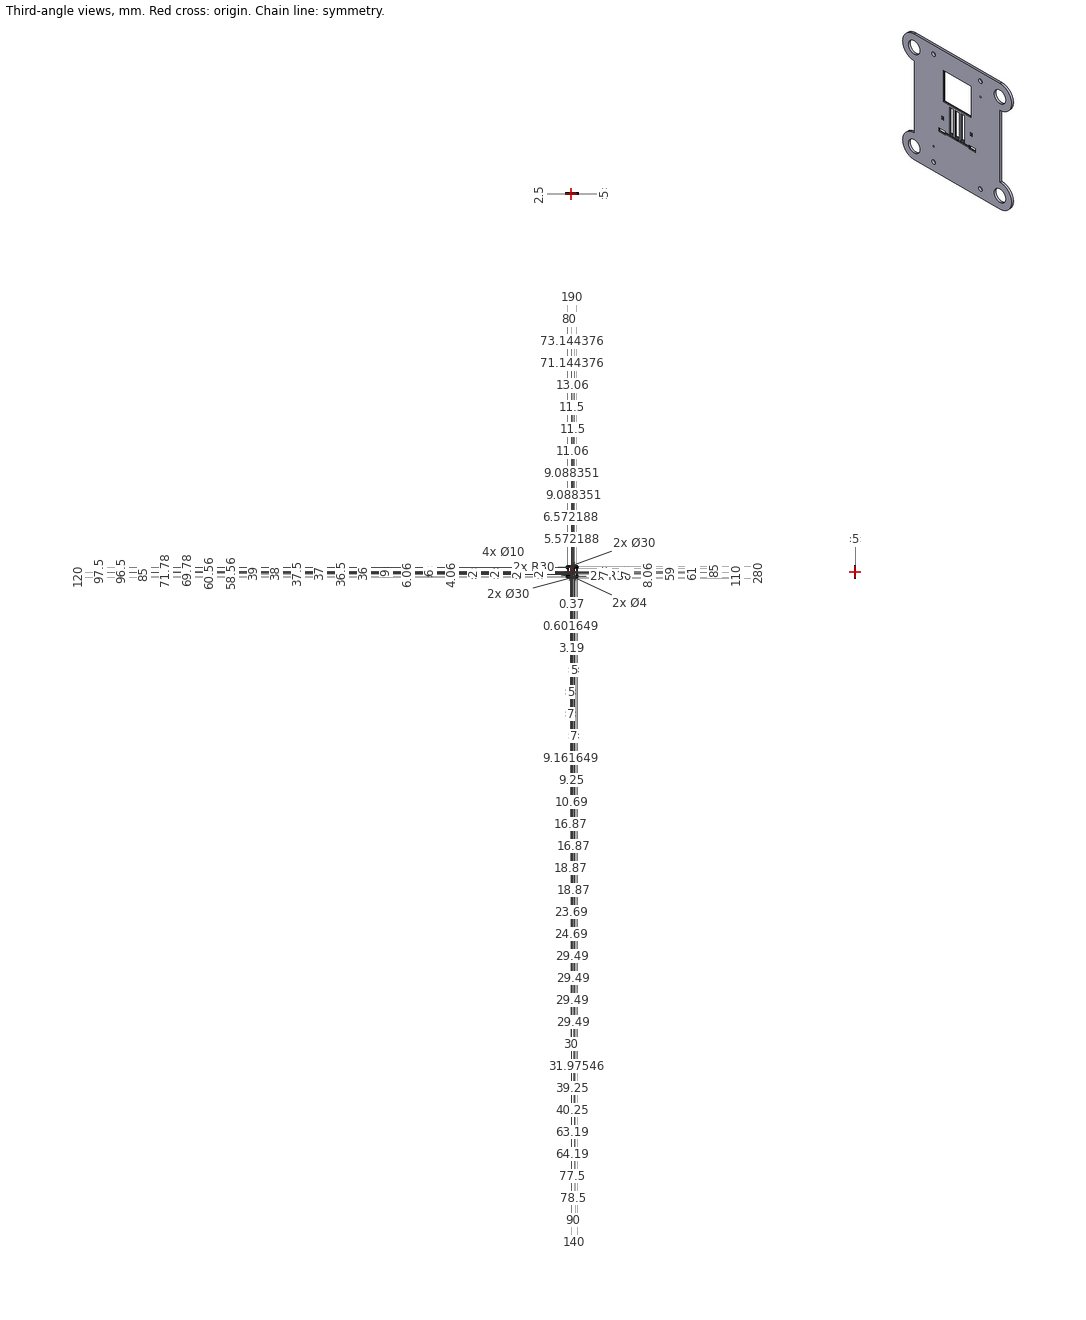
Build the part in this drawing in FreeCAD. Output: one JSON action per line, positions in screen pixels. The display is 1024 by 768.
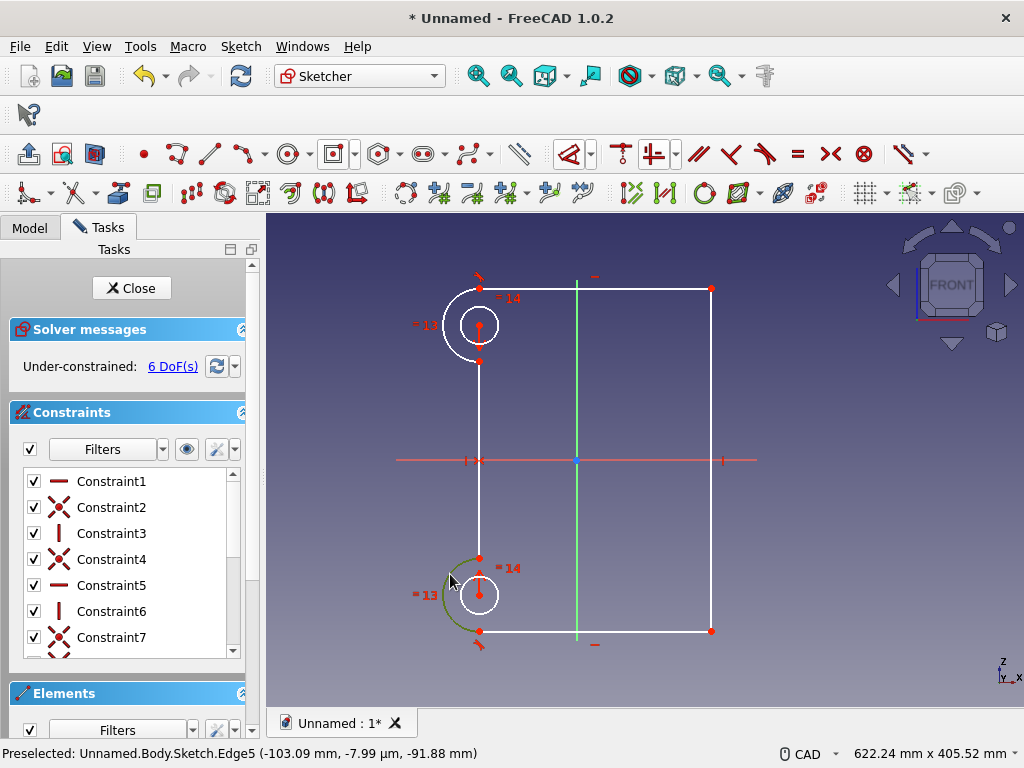
{"action": "key", "text": "k r"}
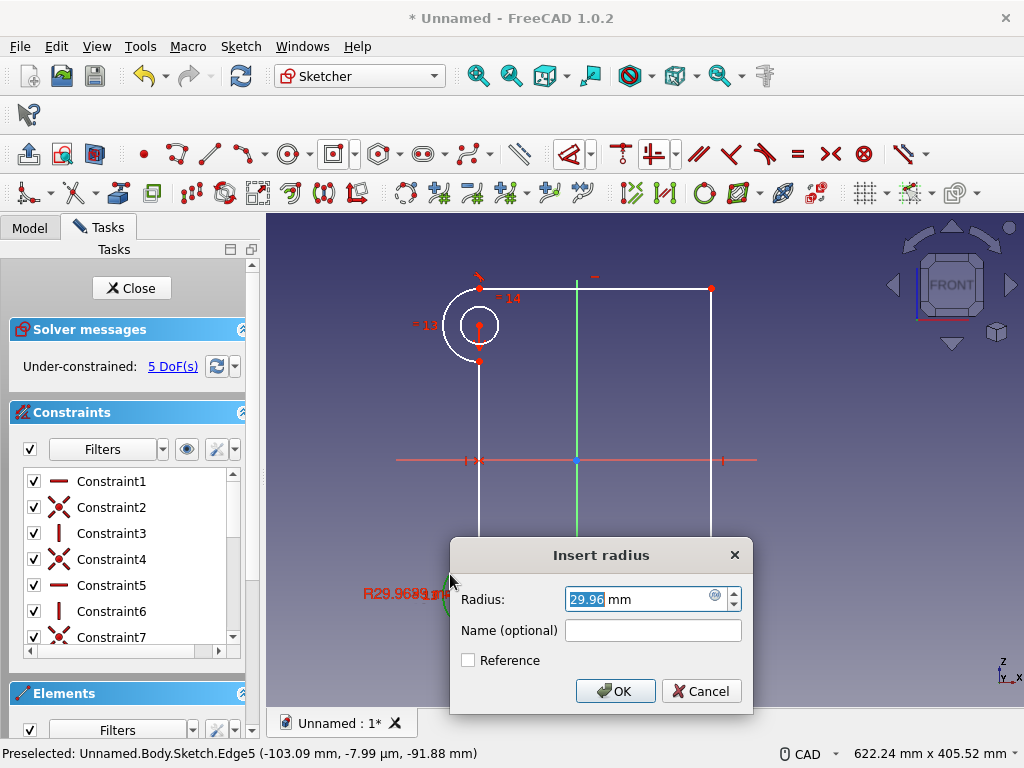
{"action": "type", "text": "30"}
{"action": "key", "text": "Return"}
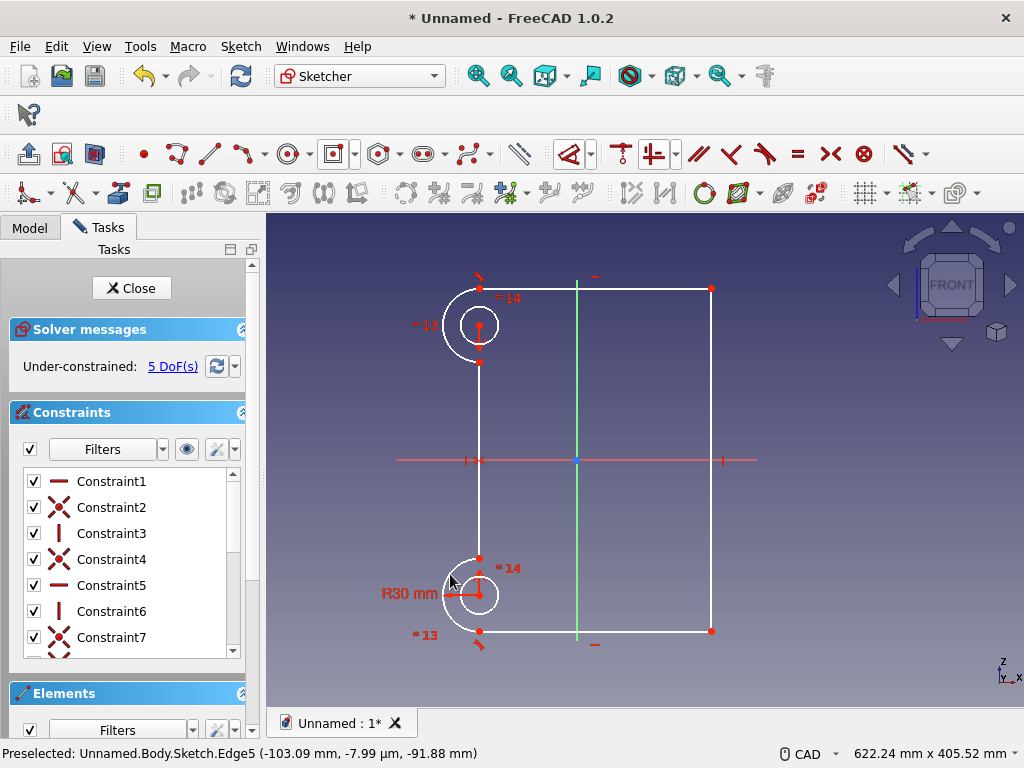
{"action": "left_click", "coordinate": [493, 312]}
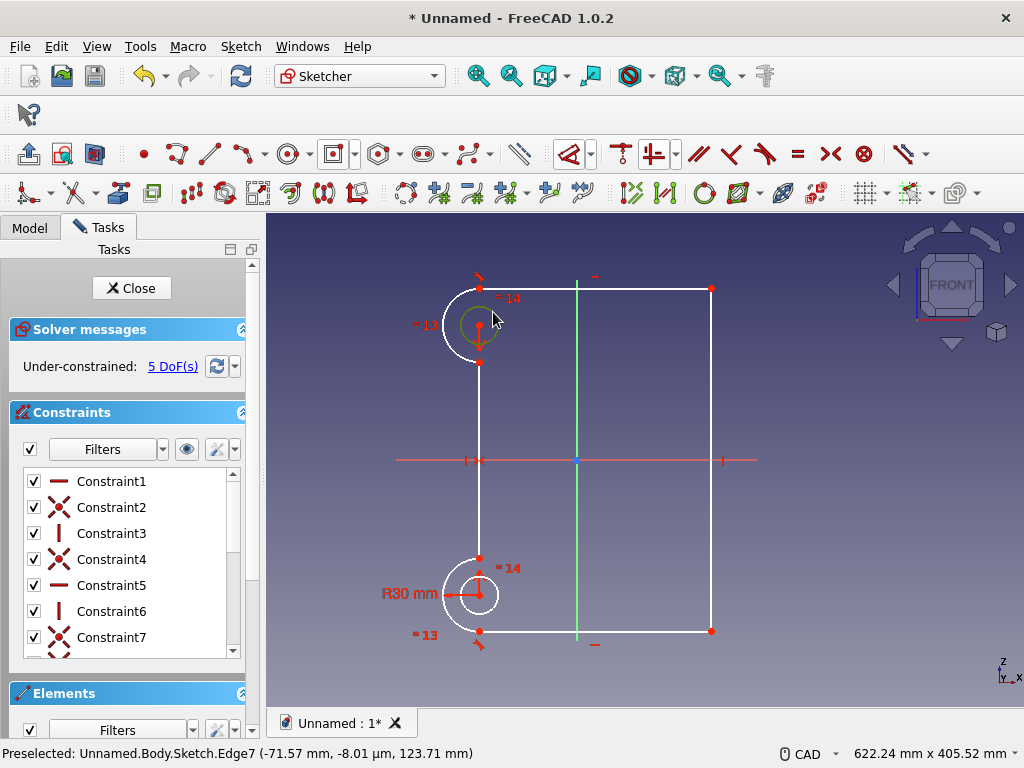
{"action": "key", "text": "k o"}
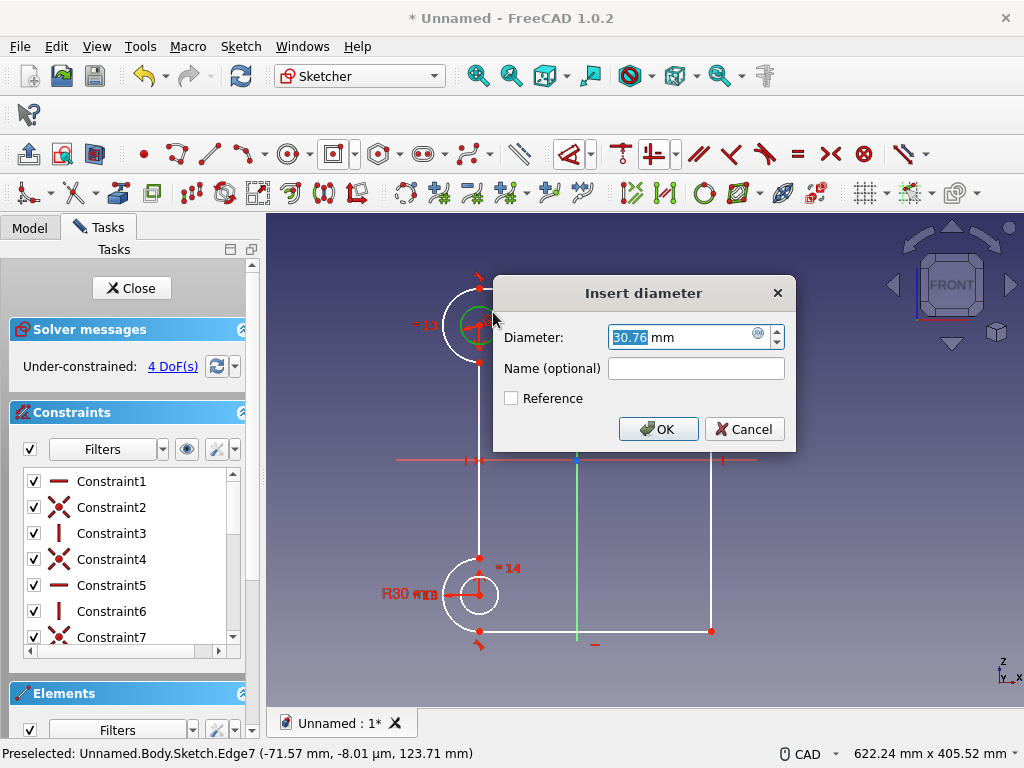
{"action": "type", "text": "30"}
{"action": "key", "text": "Return"}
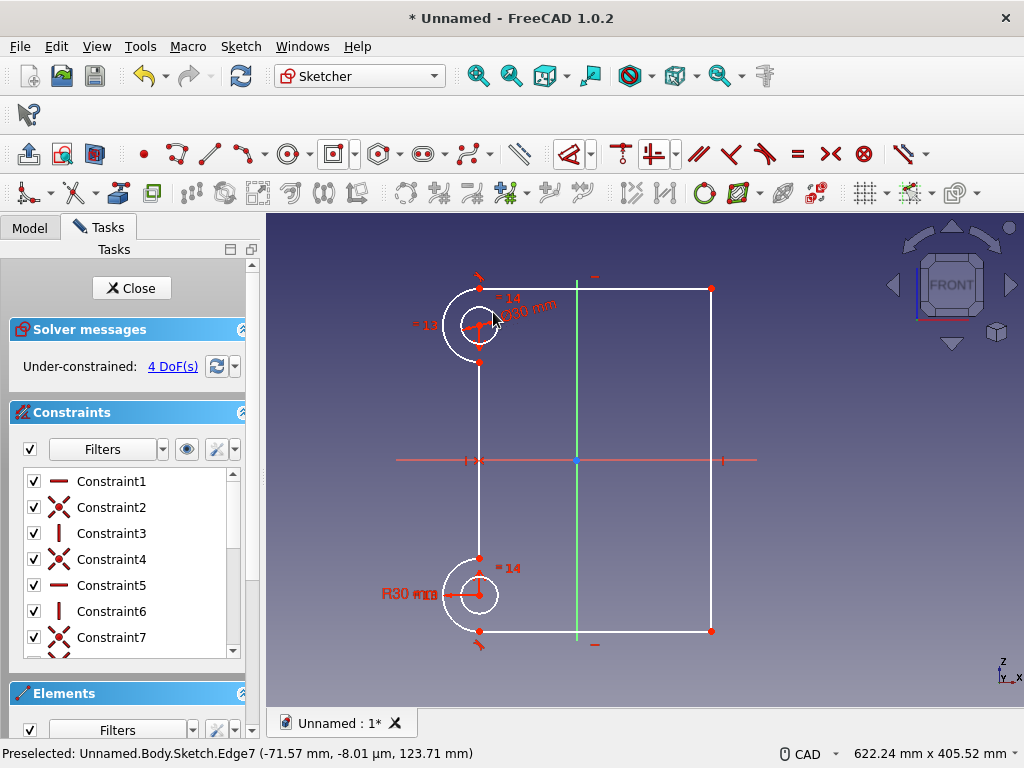
{"action": "left_click", "coordinate": [479, 325]}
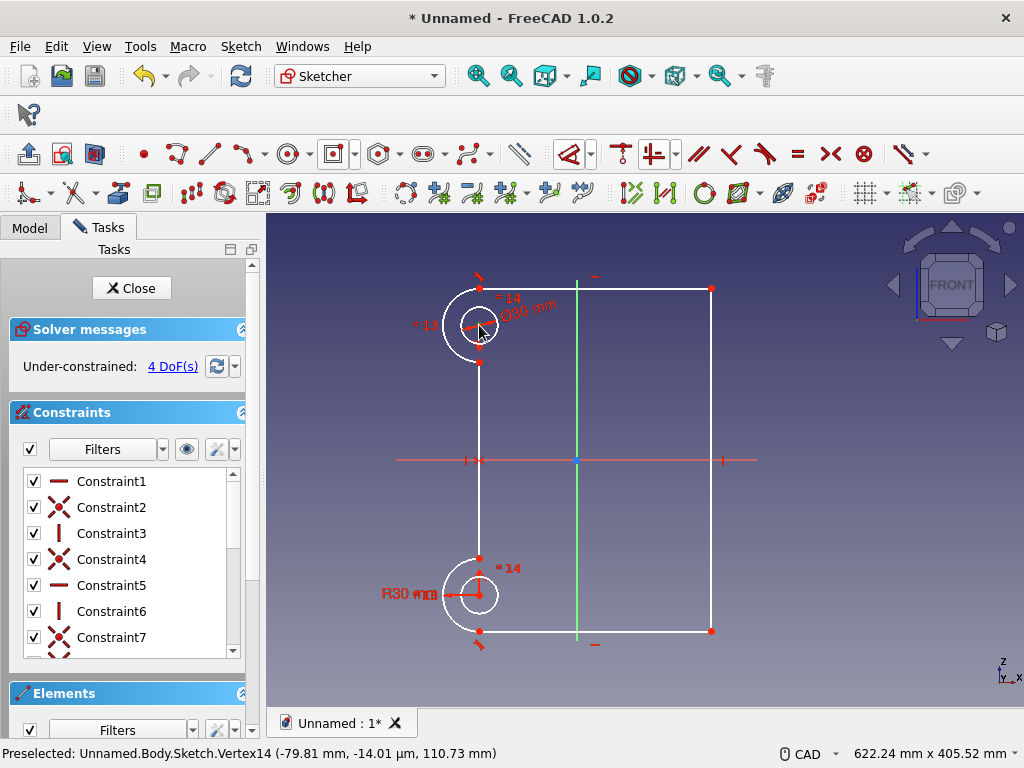
{"action": "key", "text": "l"}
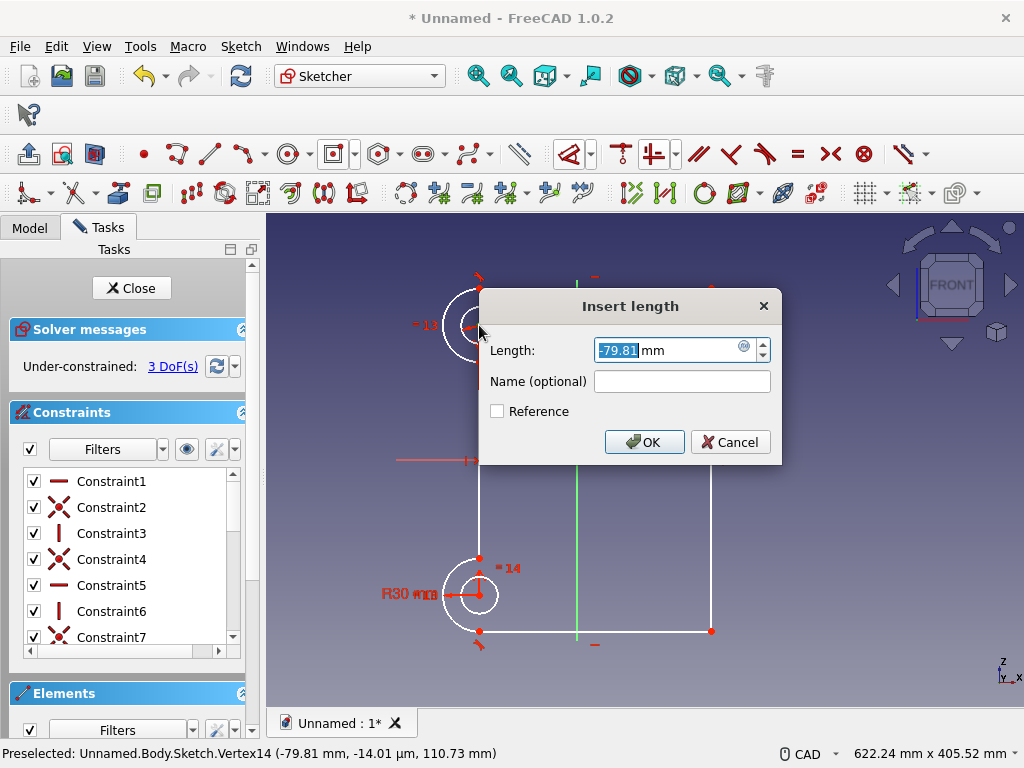
{"action": "type", "text": "-80"}
{"action": "key", "text": "Return"}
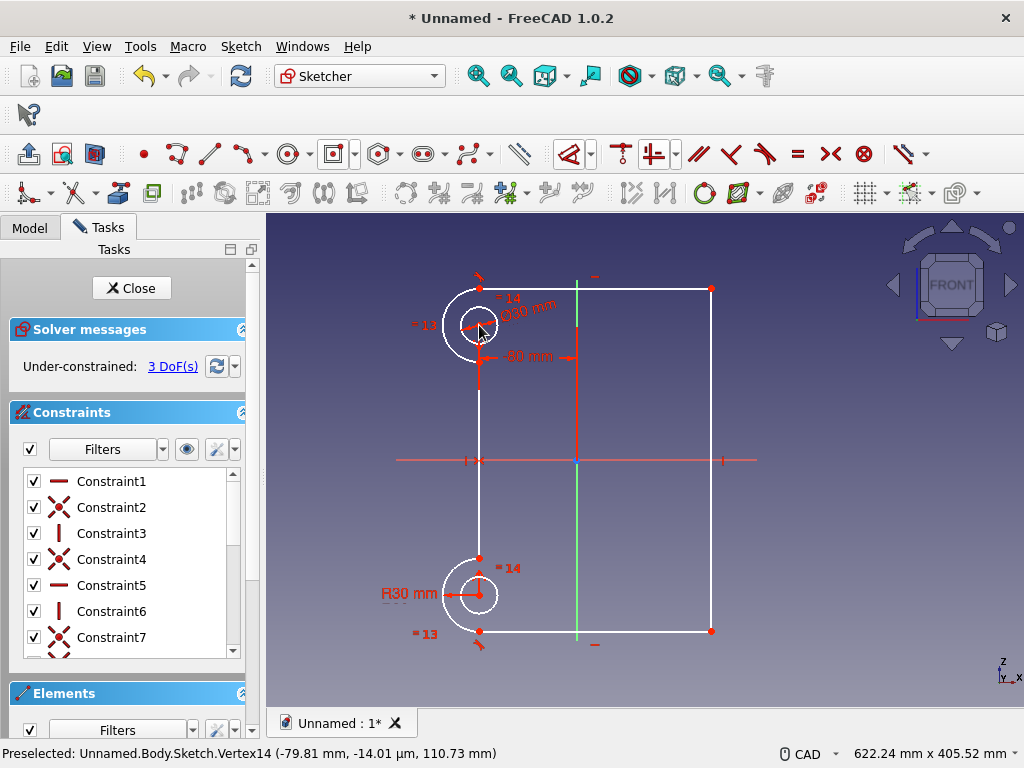
{"action": "left_click", "coordinate": [549, 289]}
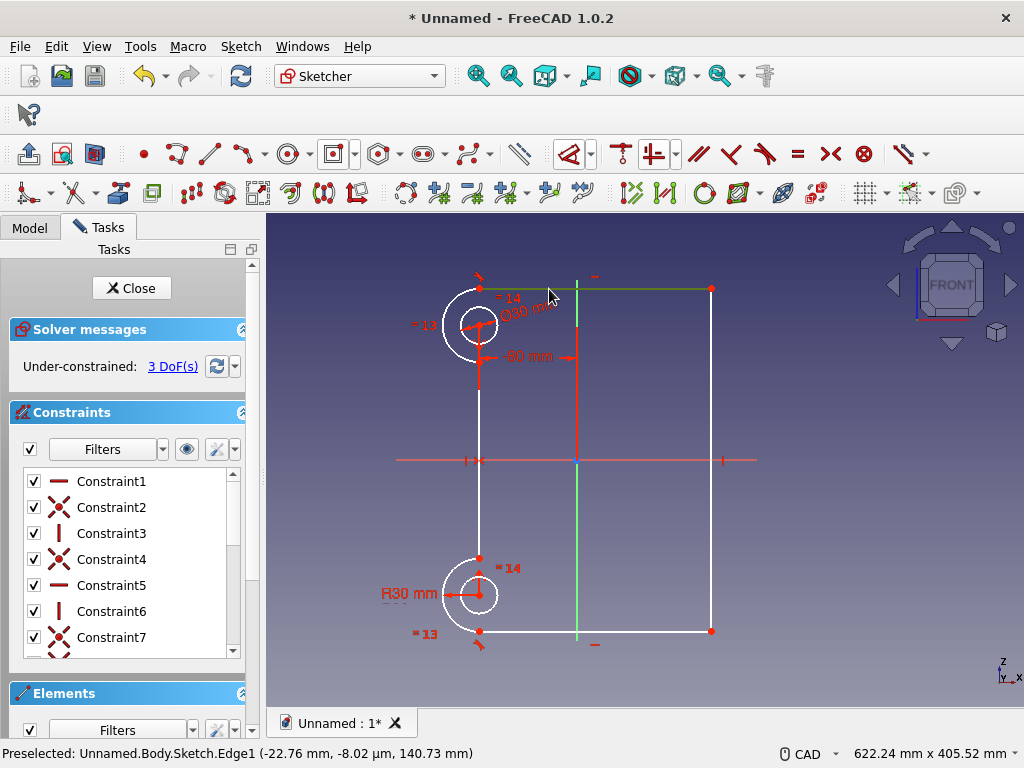
{"action": "left_click", "coordinate": [590, 154]}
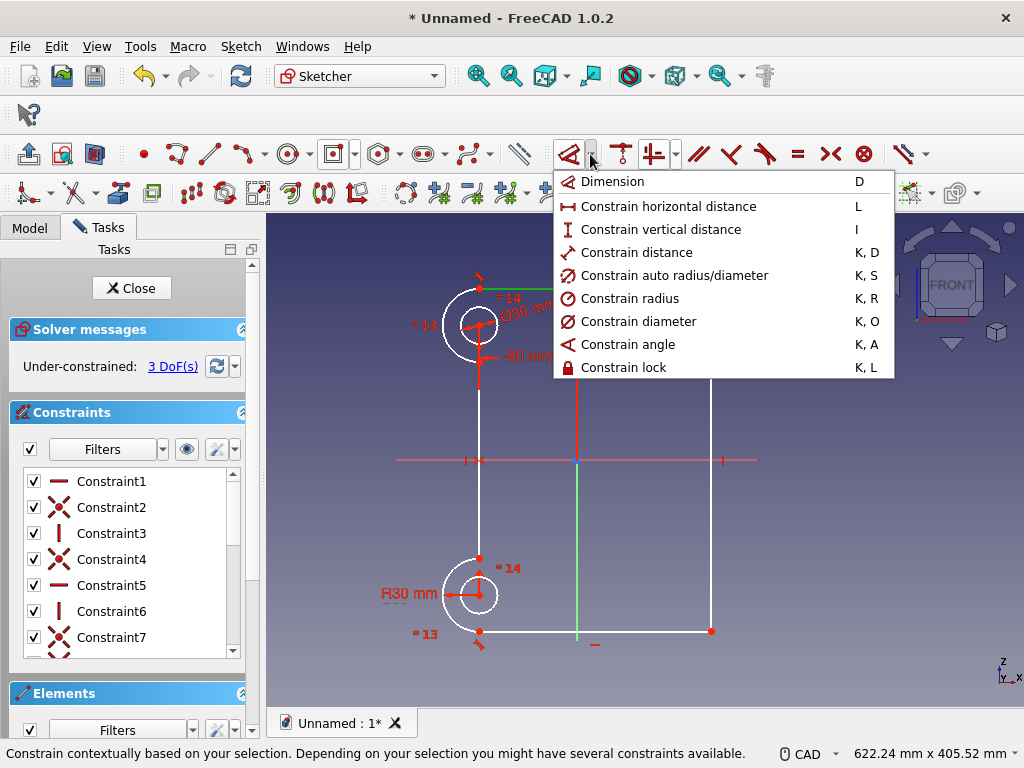
{"action": "left_click", "coordinate": [724, 206]}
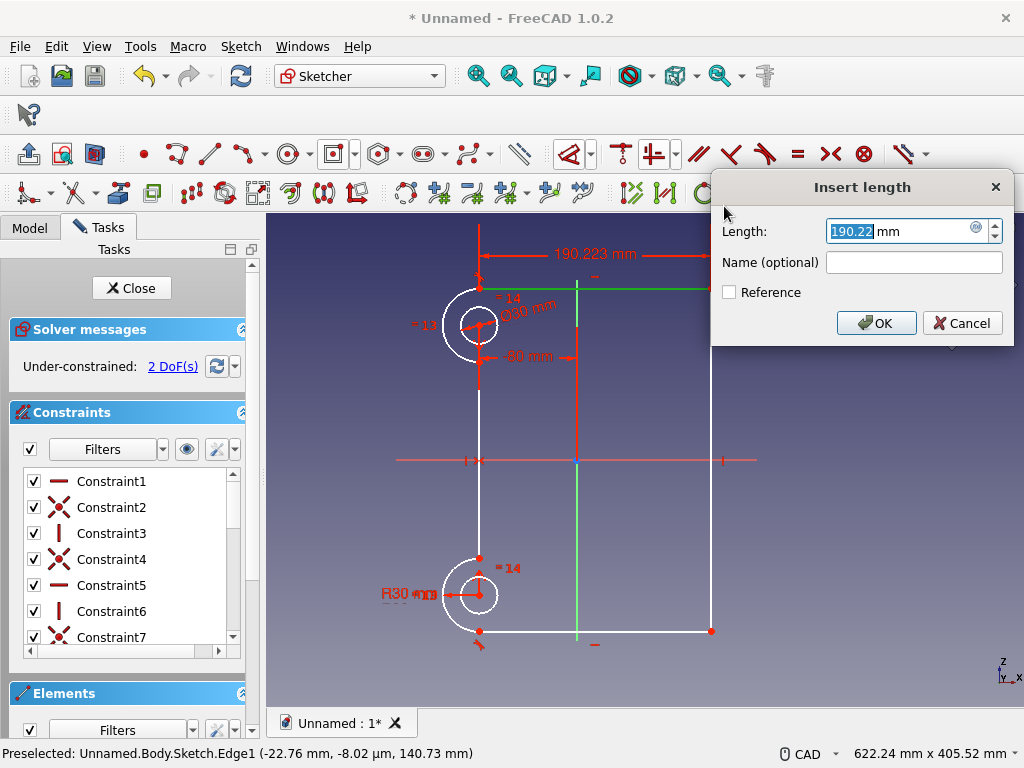
{"action": "type", "text": "190"}
{"action": "key", "text": "Return"}